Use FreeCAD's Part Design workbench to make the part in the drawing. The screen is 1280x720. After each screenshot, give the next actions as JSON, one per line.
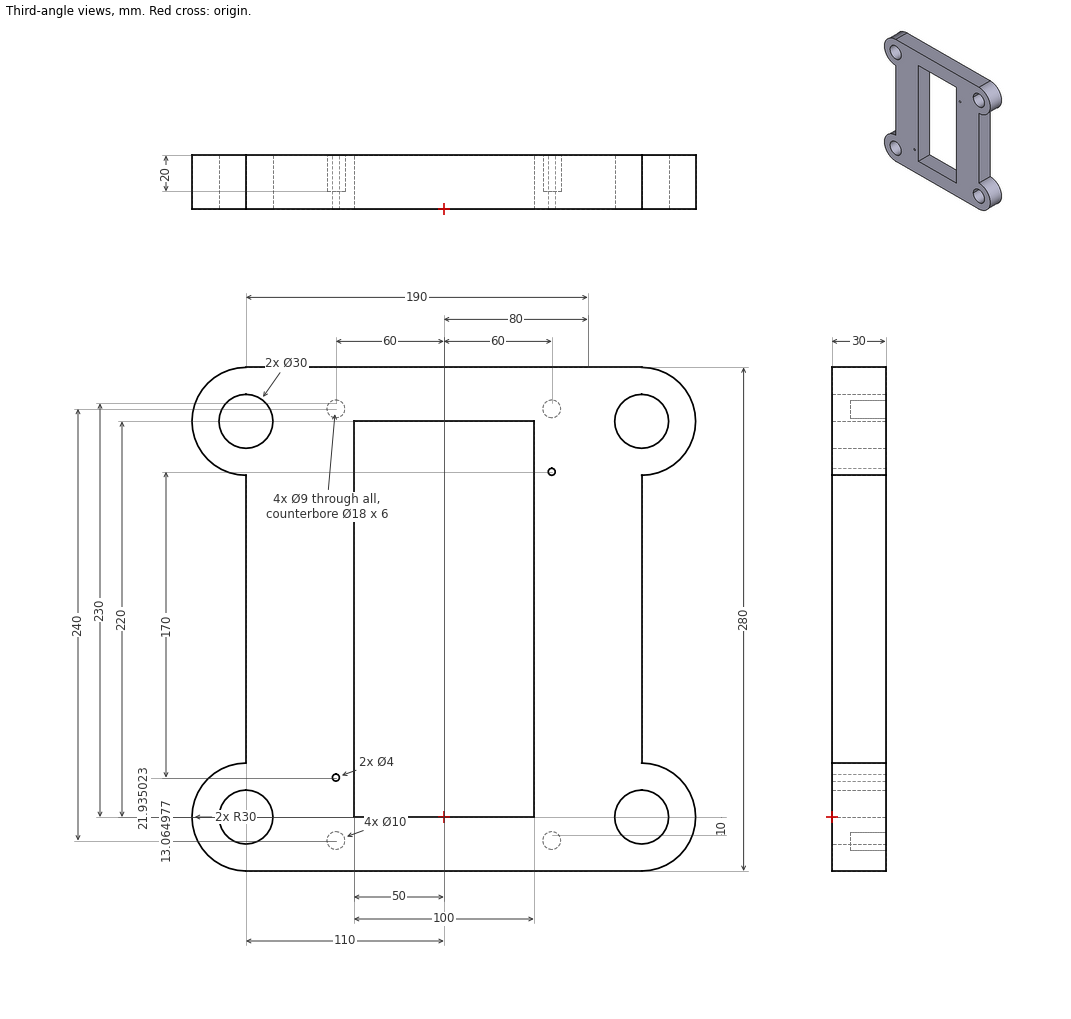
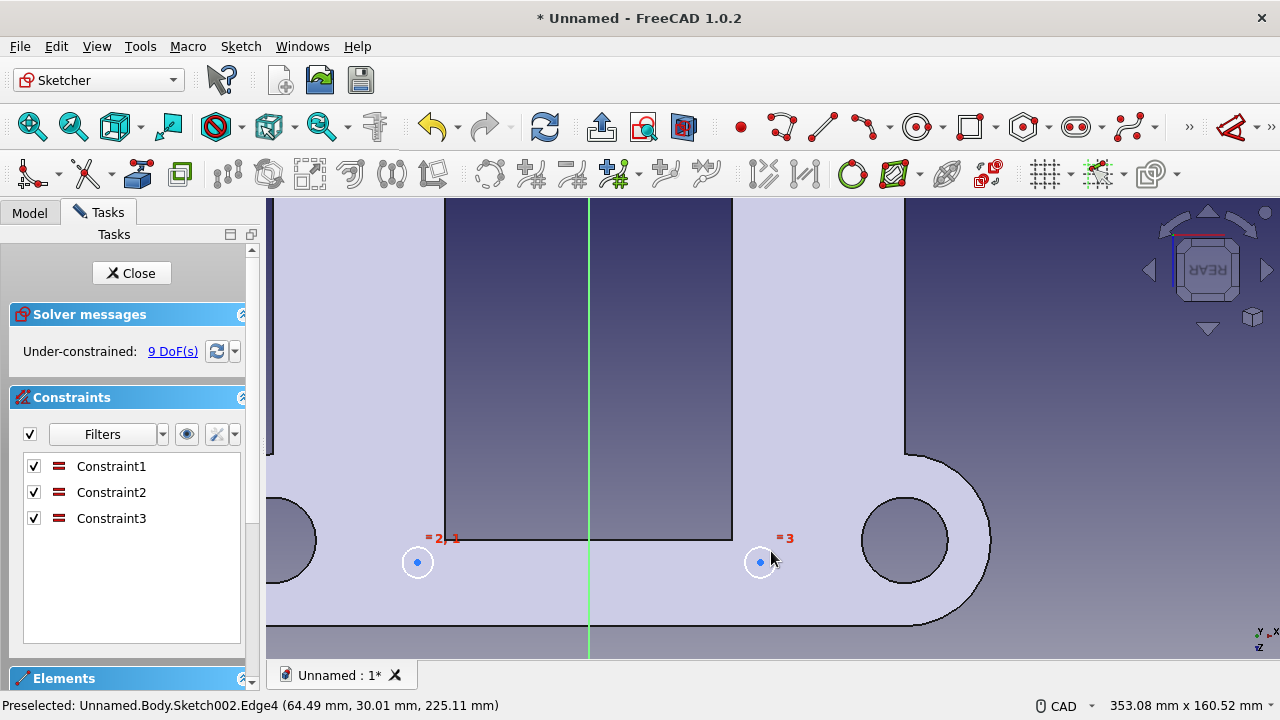
{"action": "key", "text": "d"}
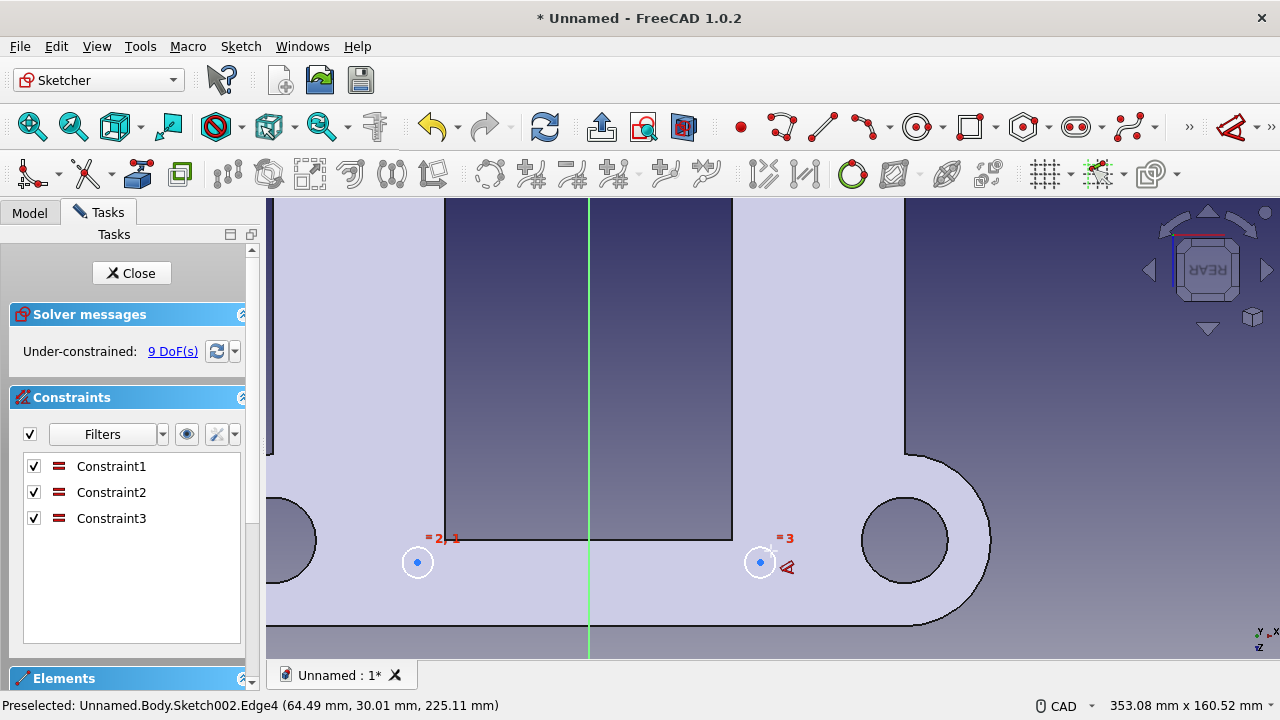
{"action": "scroll", "coordinate": [772, 552], "scroll_direction": "down", "scroll_amount": 5}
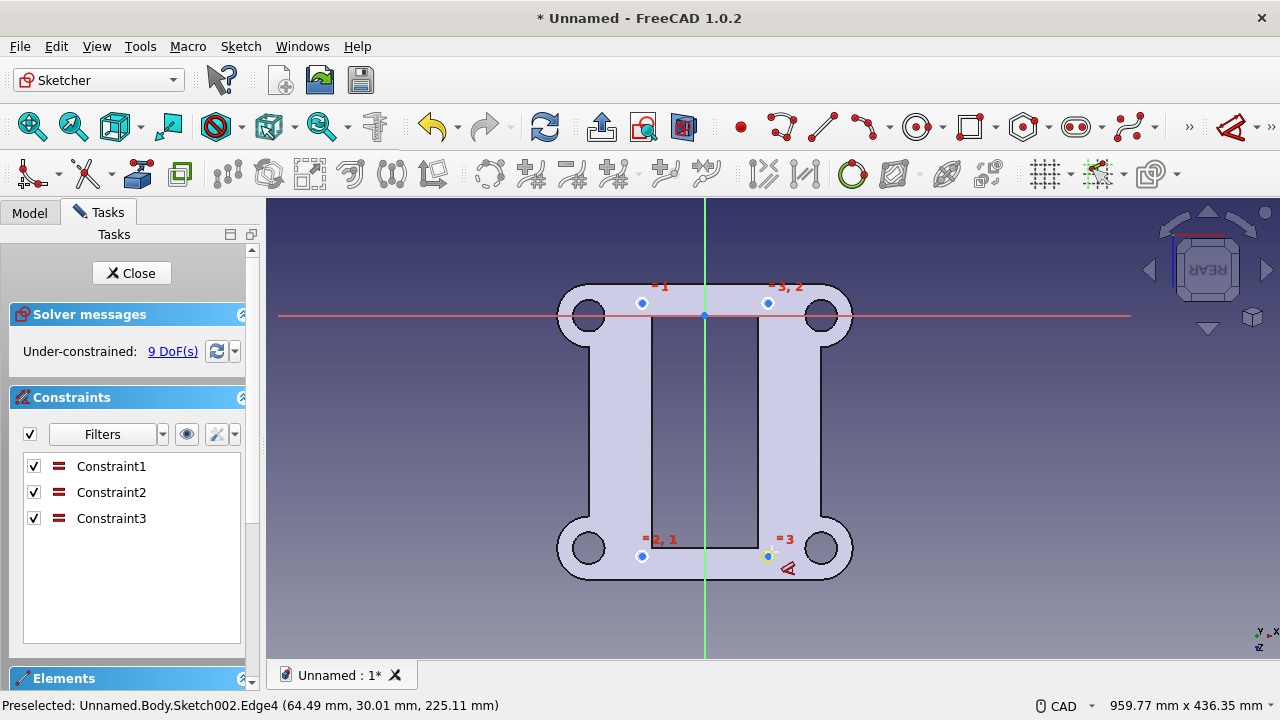
{"action": "scroll", "coordinate": [646, 299], "scroll_direction": "up", "scroll_amount": 7}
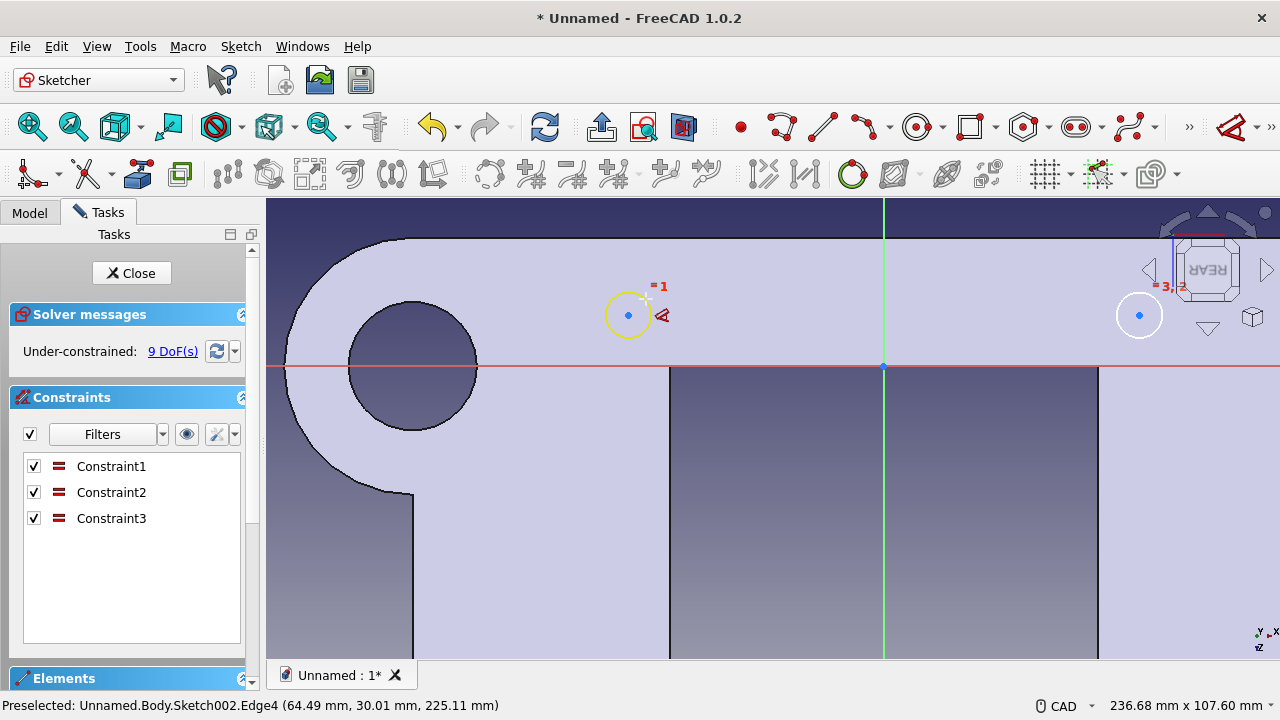
{"action": "left_click", "coordinate": [645, 299]}
{"action": "left_click", "coordinate": [668, 276]}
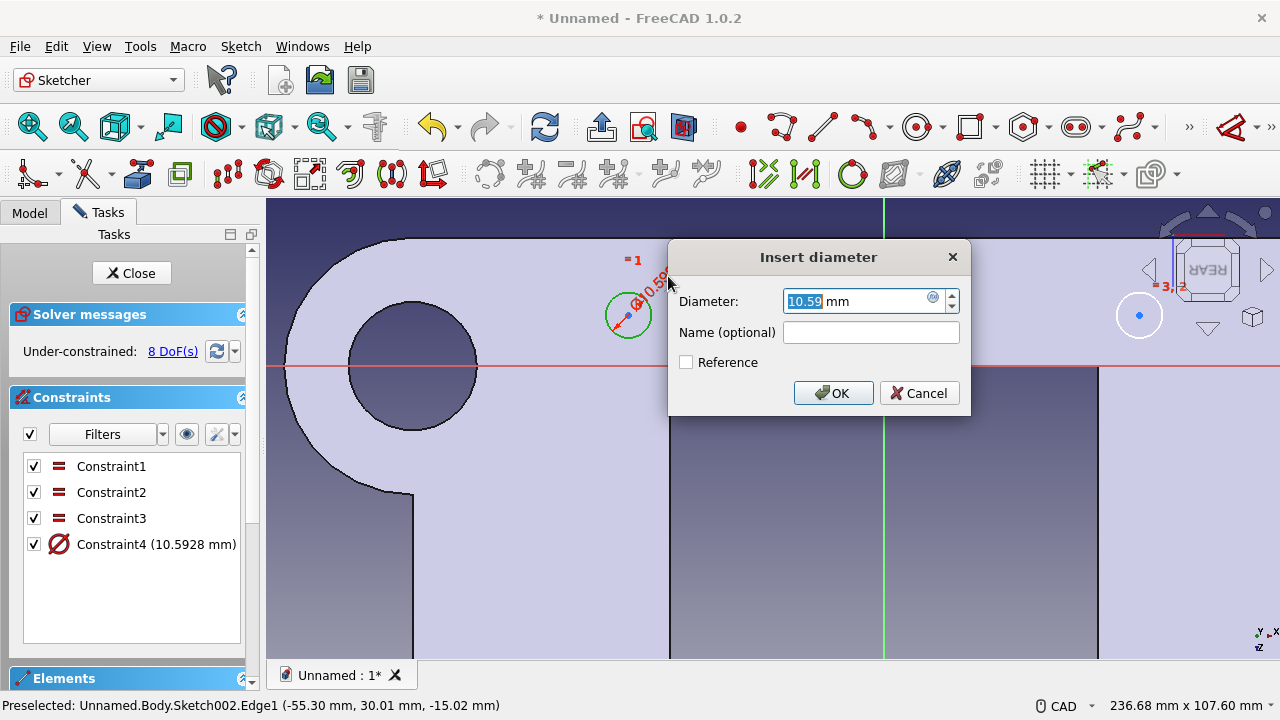
{"action": "type", "text": "10"}
{"action": "key", "text": "Return"}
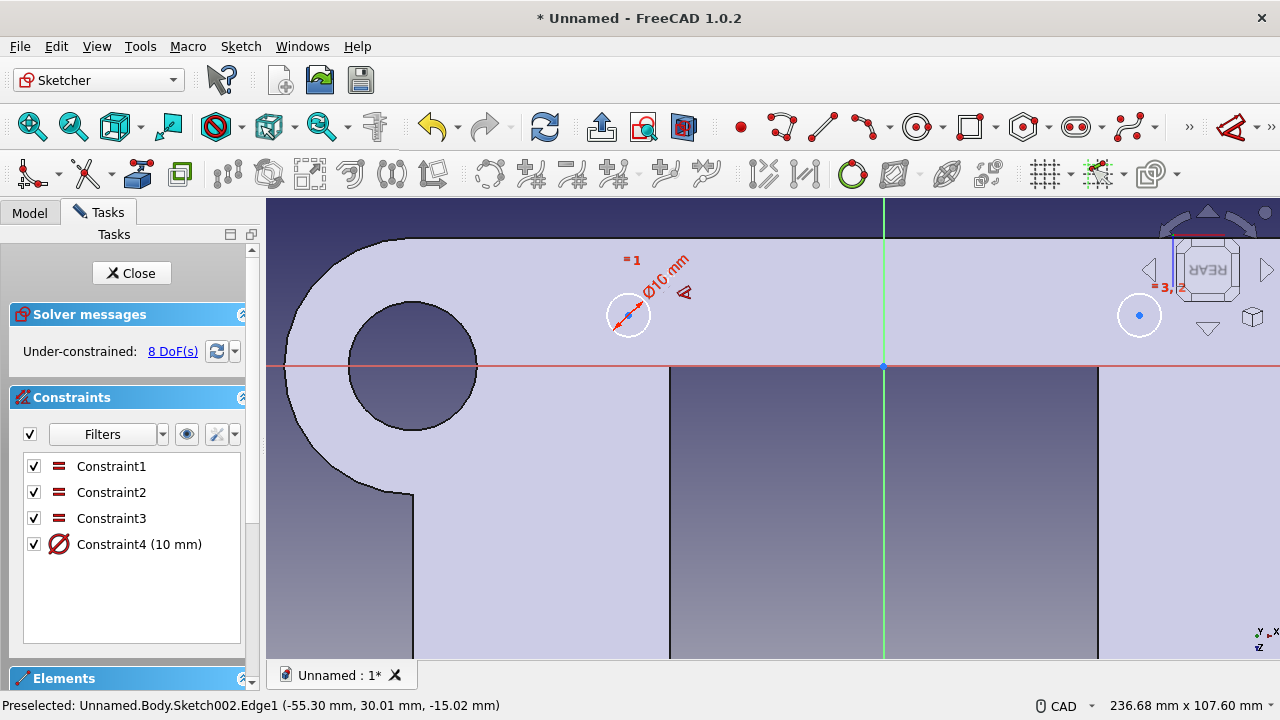
{"action": "left_click", "coordinate": [629, 315]}
{"action": "left_click", "coordinate": [756, 281]}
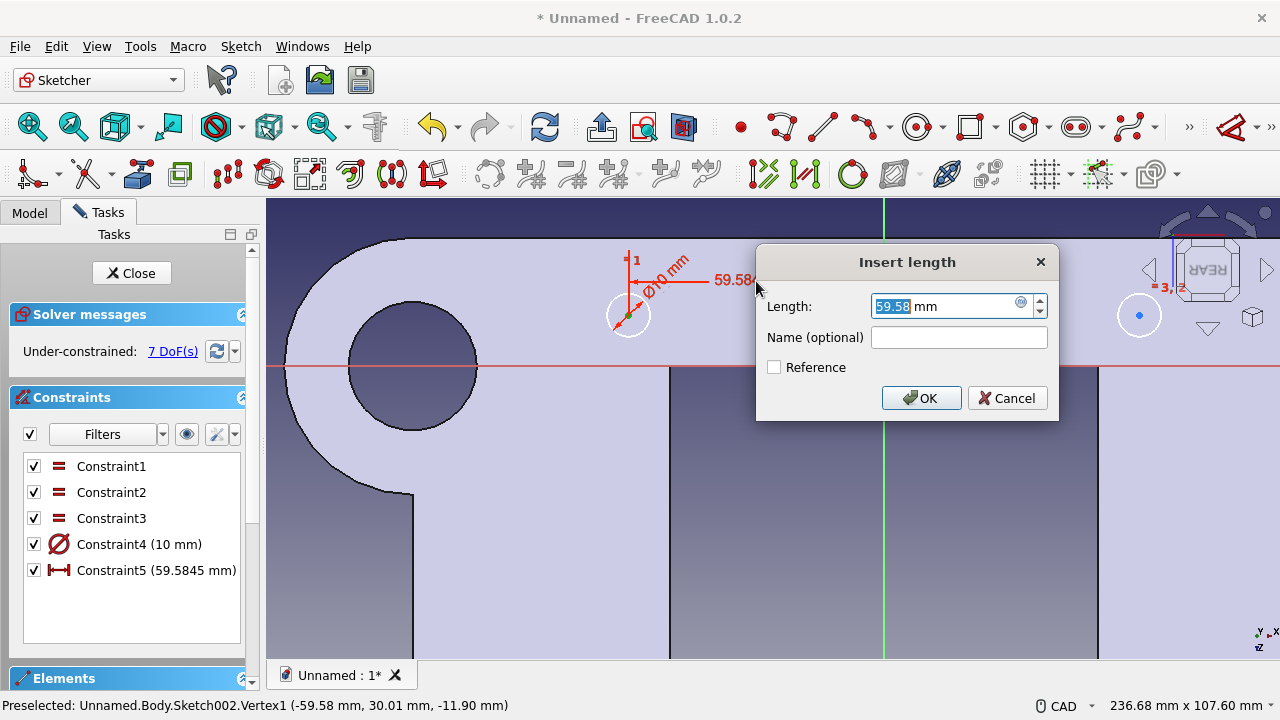
{"action": "type", "text": "60"}
{"action": "key", "text": "Return"}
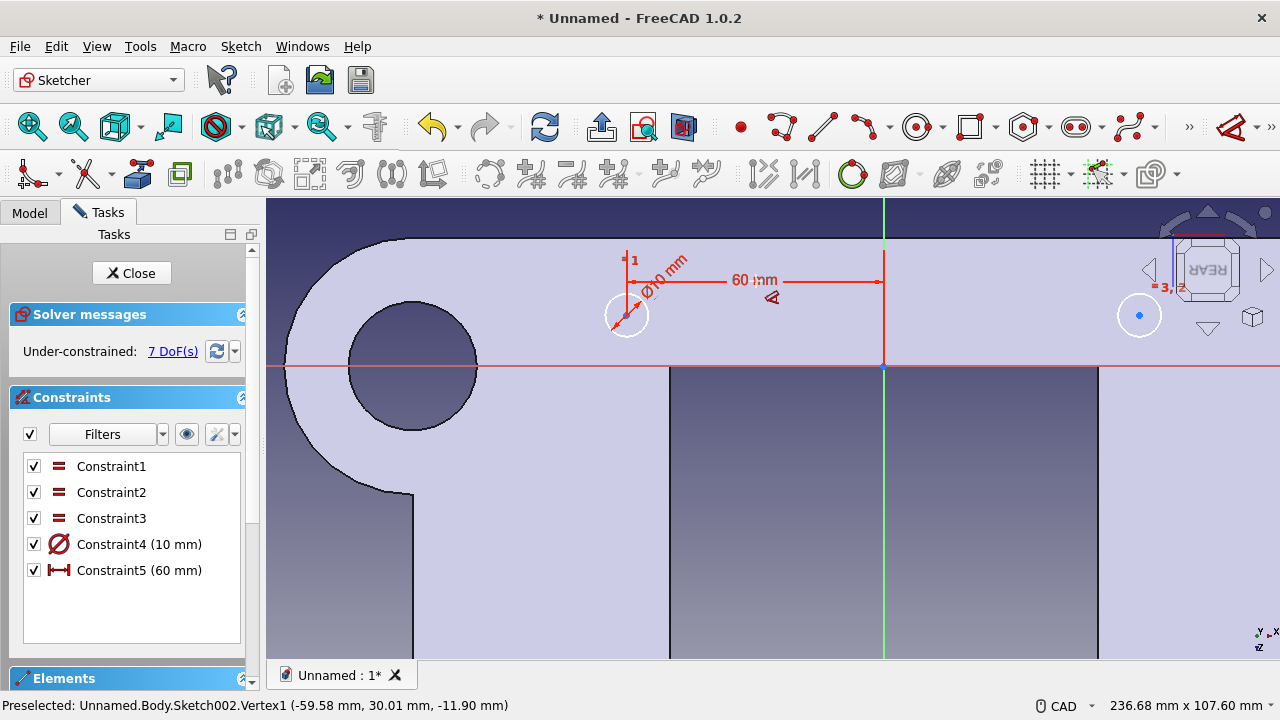
{"action": "scroll", "coordinate": [646, 299], "scroll_direction": "down", "scroll_amount": 7}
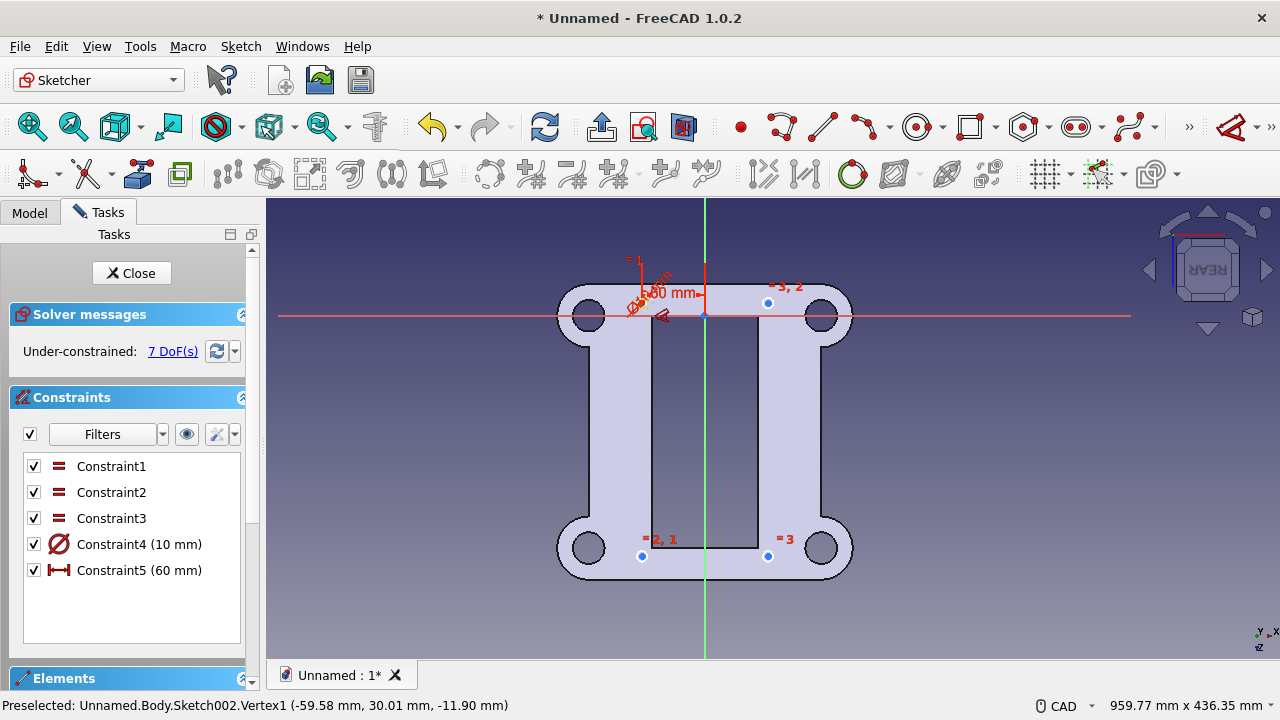
{"action": "left_click", "coordinate": [642, 556]}
{"action": "left_click", "coordinate": [673, 590]}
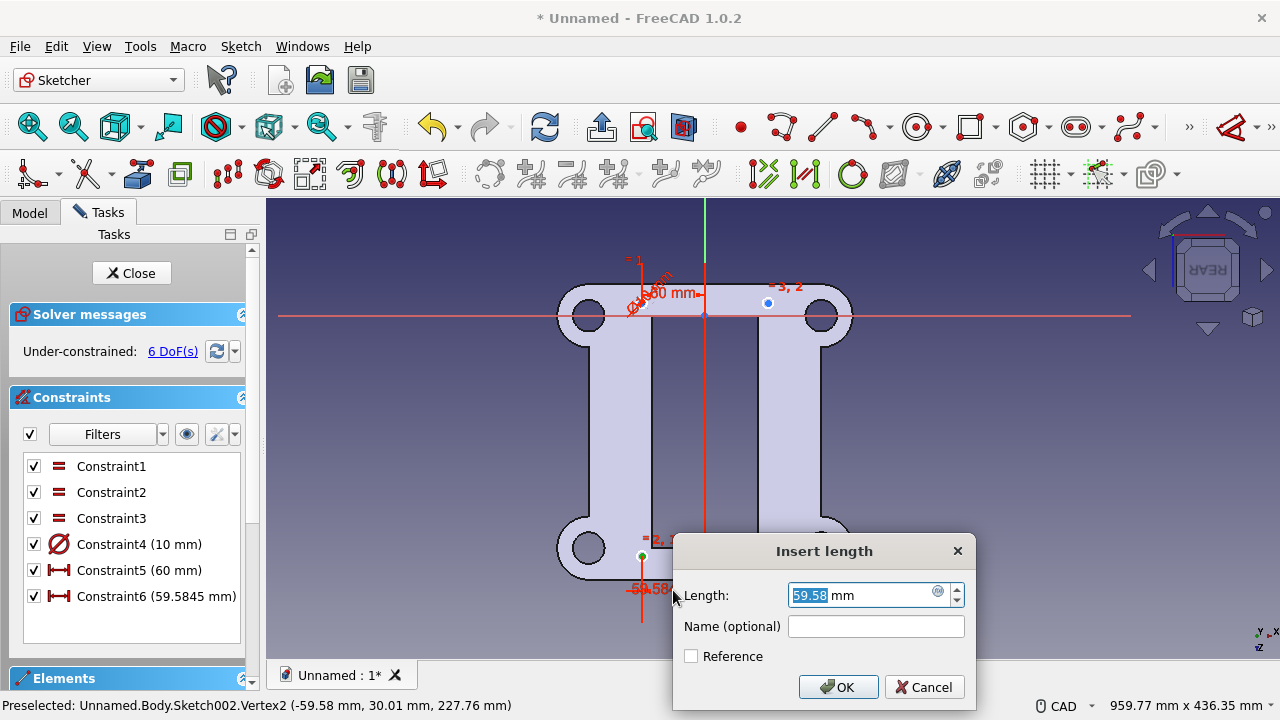
{"action": "type", "text": "60"}
{"action": "key", "text": "Return"}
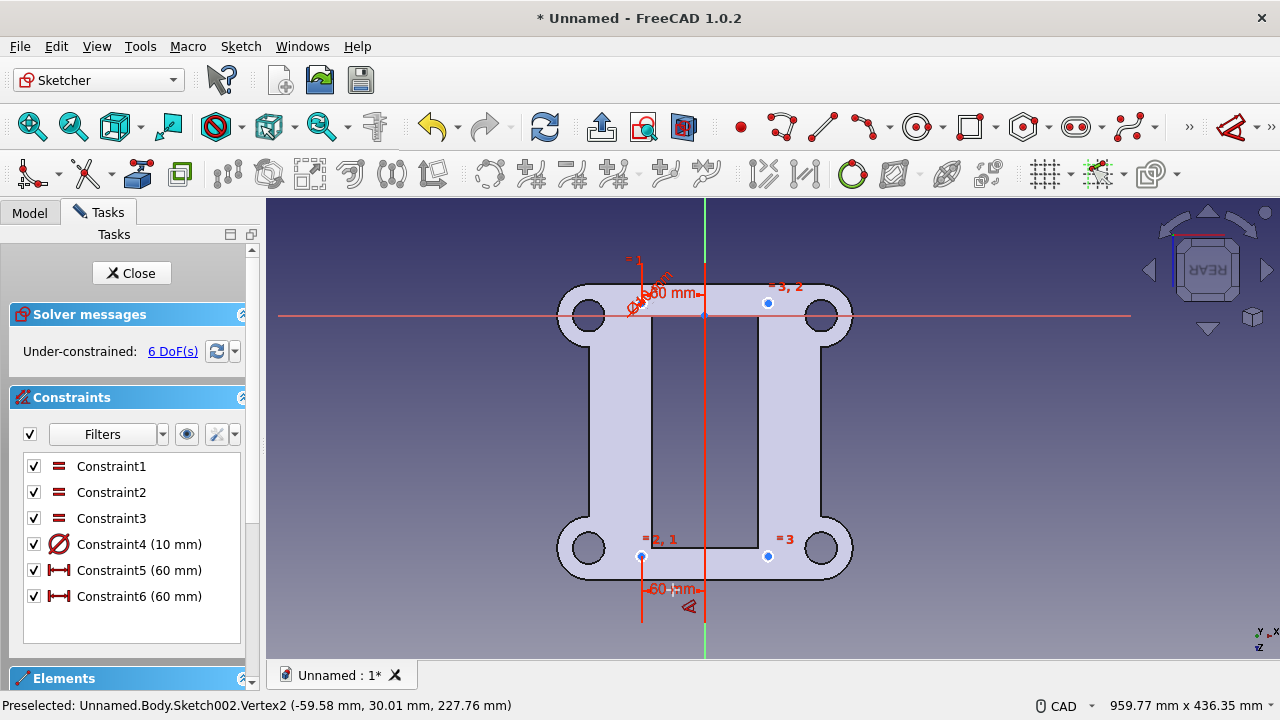
{"action": "left_click", "coordinate": [768, 303]}
{"action": "left_click", "coordinate": [736, 269]}